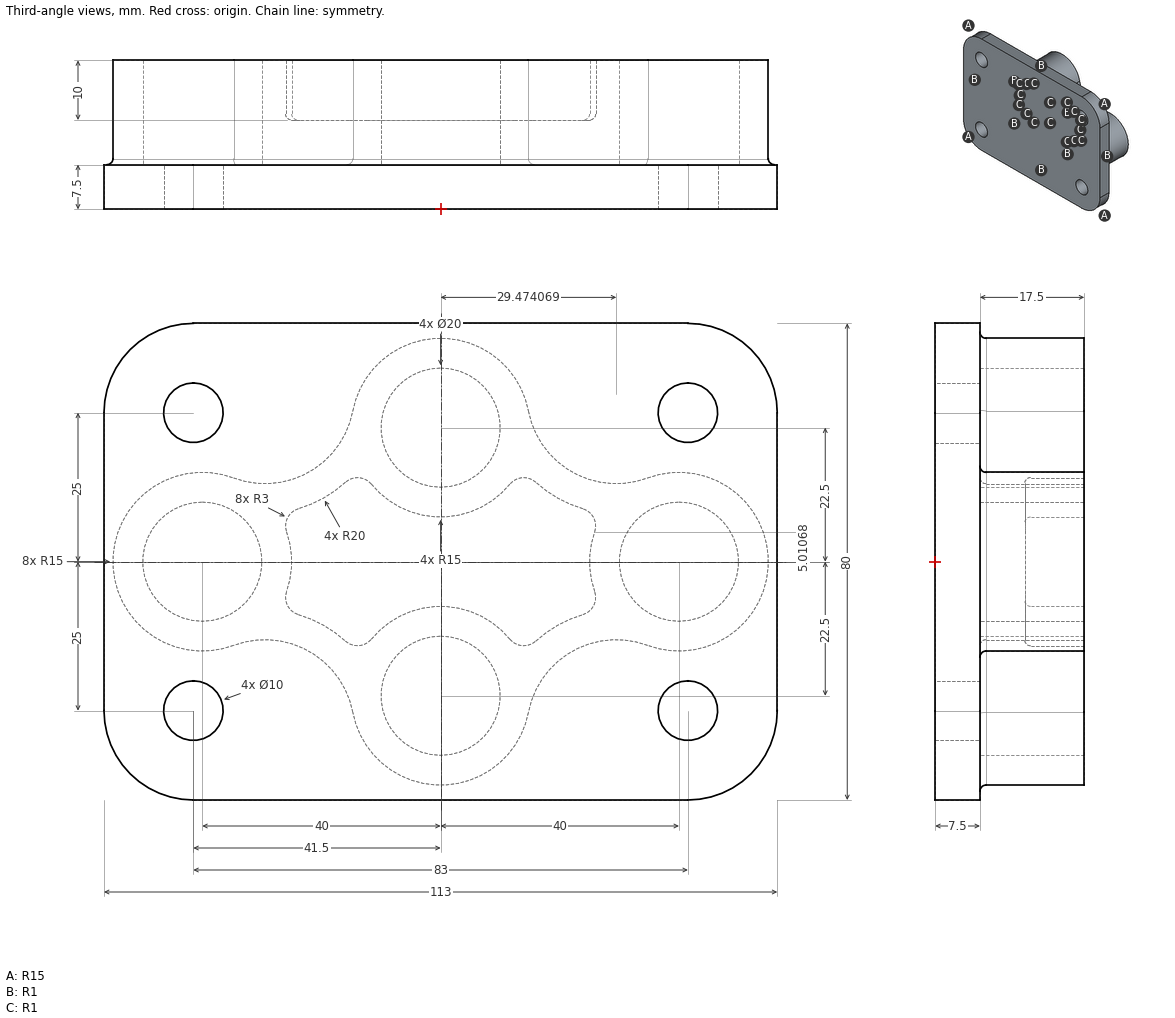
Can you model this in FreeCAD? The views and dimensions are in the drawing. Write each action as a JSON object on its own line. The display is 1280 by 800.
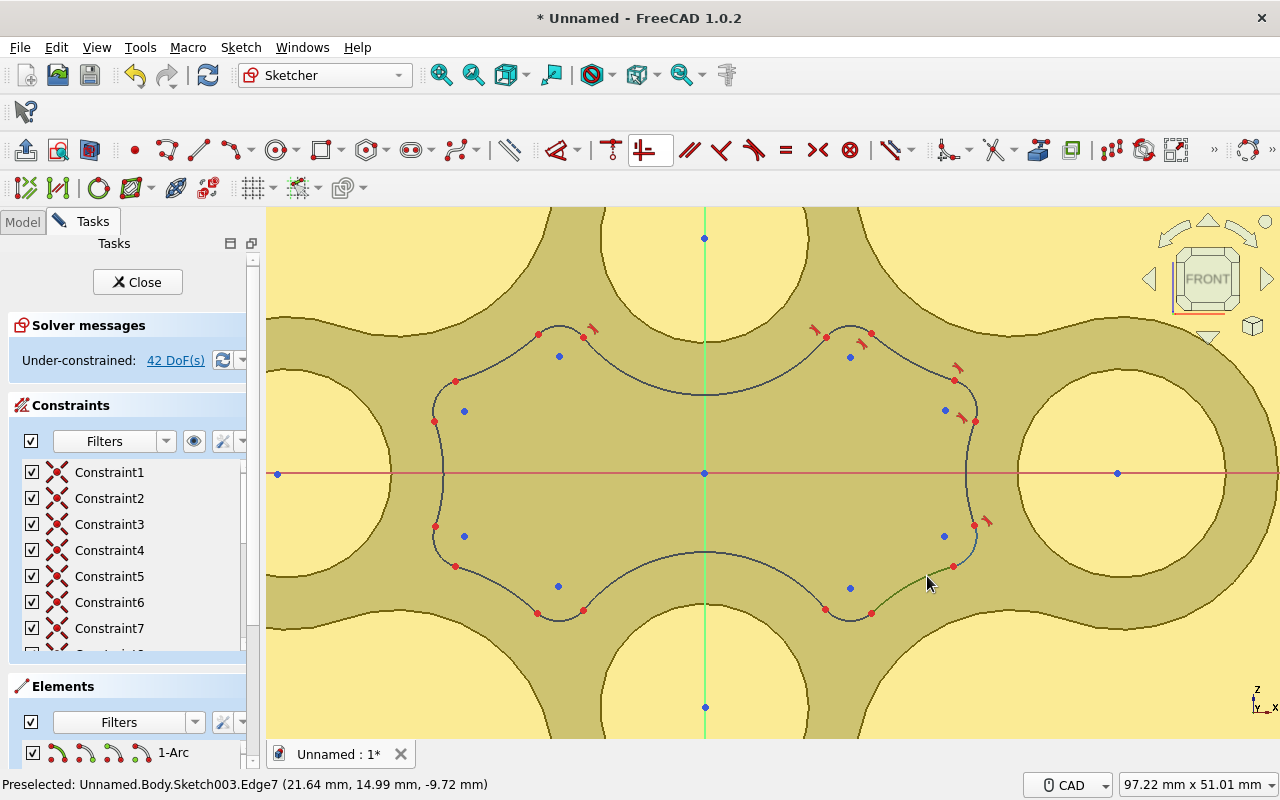
{"action": "key", "text": "t"}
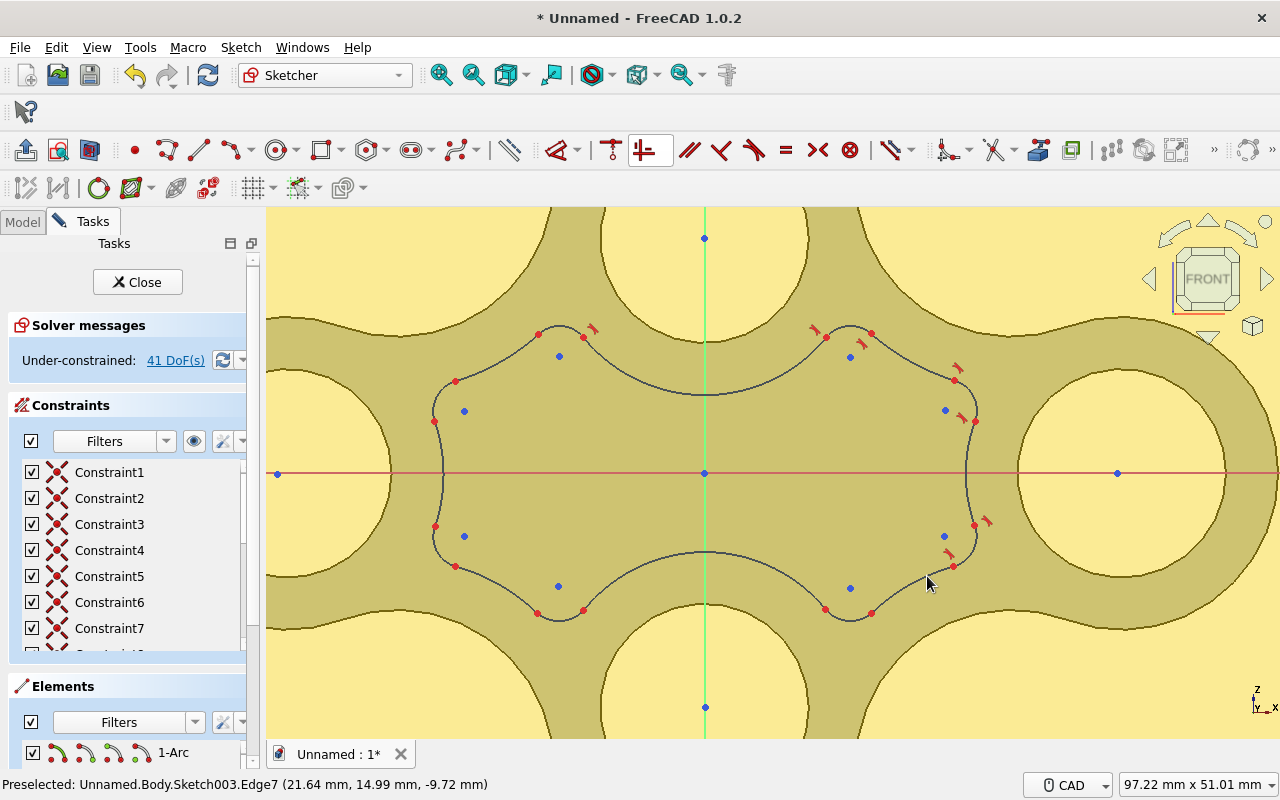
{"action": "left_click", "coordinate": [927, 576]}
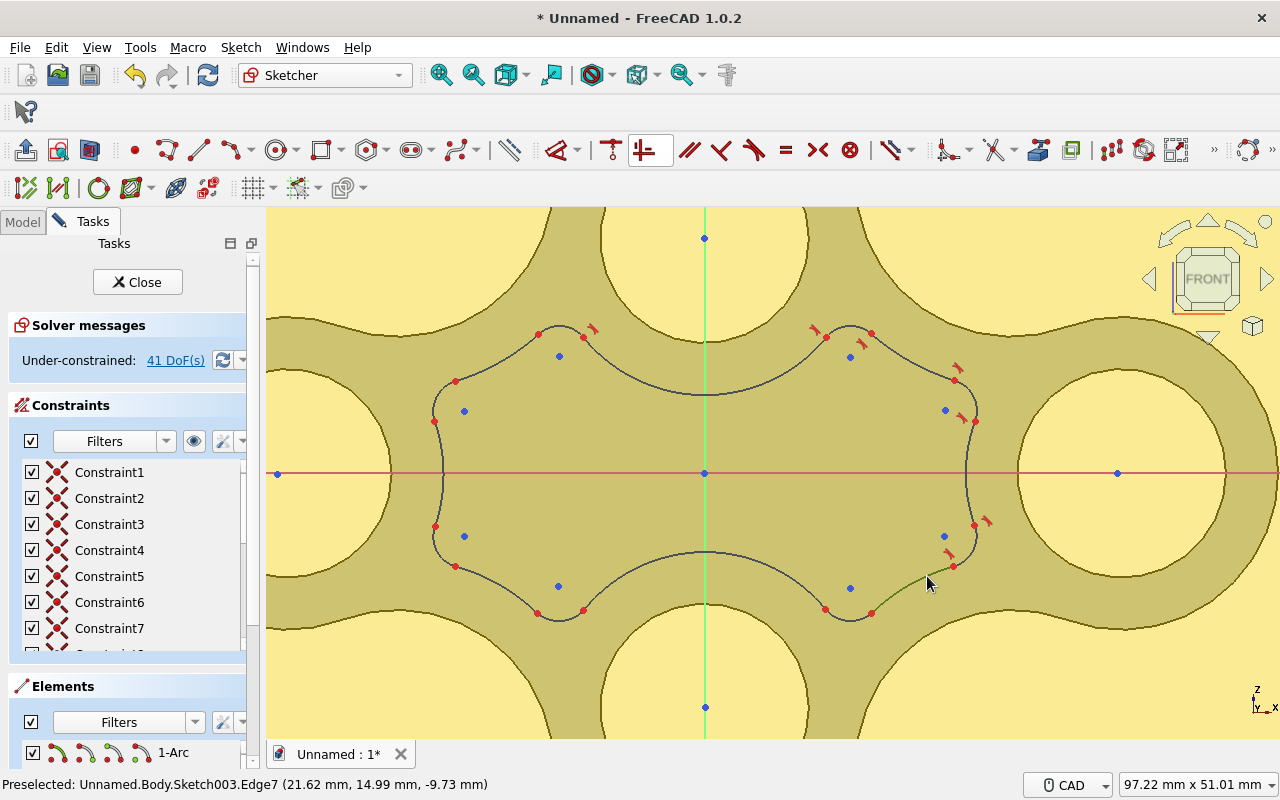
{"action": "left_click", "coordinate": [838, 618]}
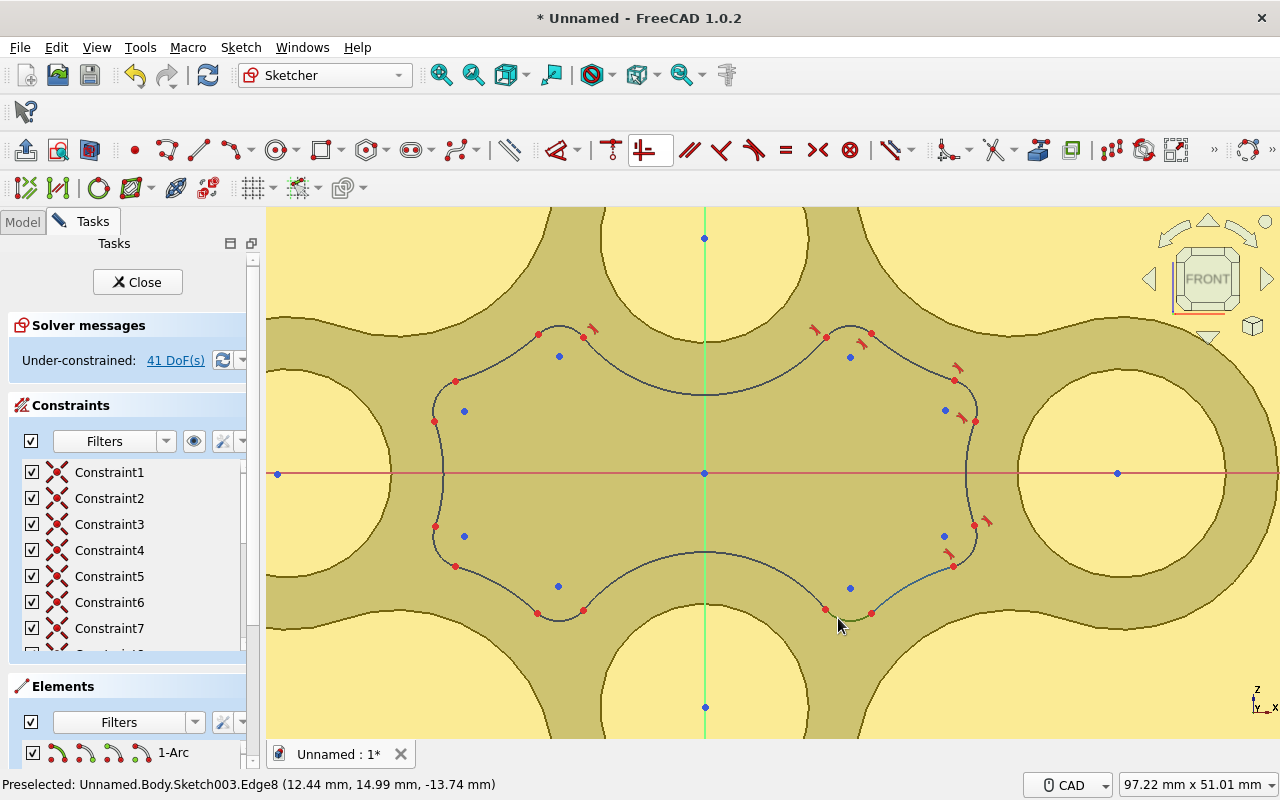
{"action": "key", "text": "t"}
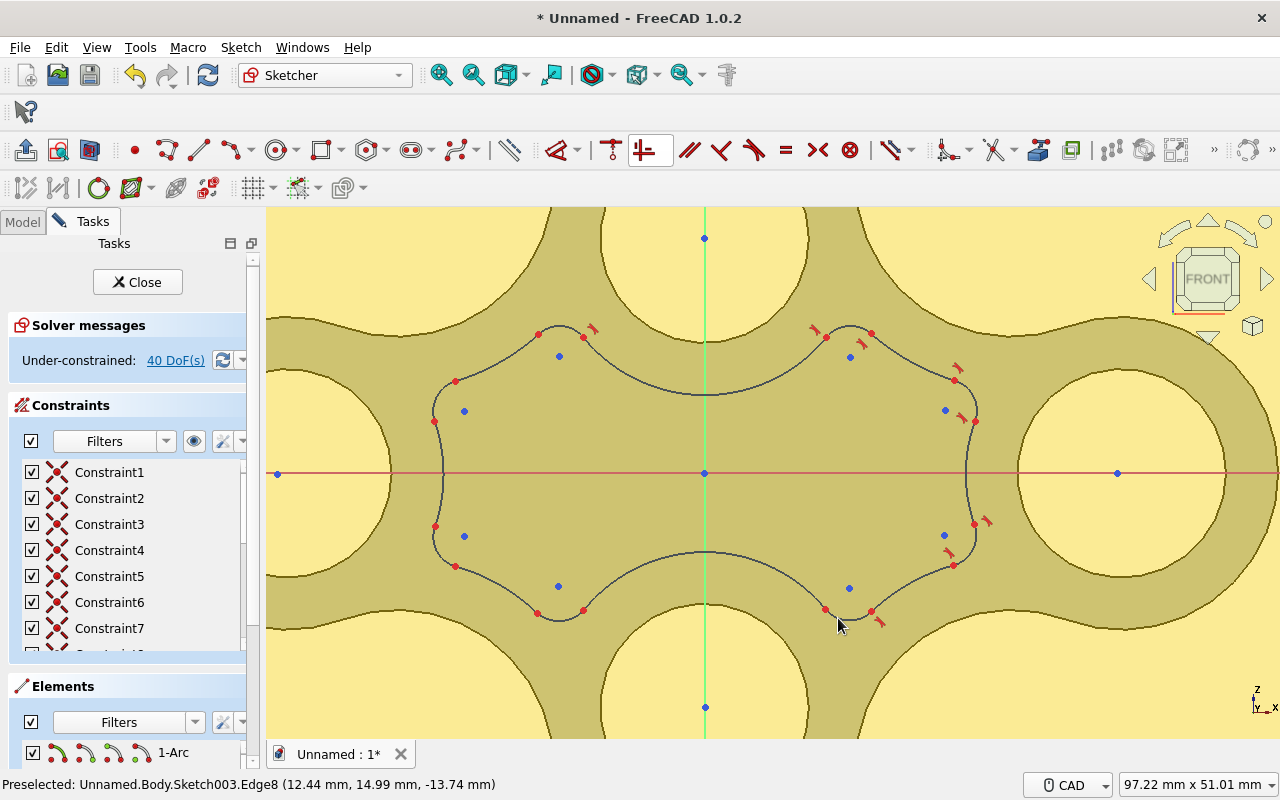
{"action": "left_click", "coordinate": [838, 618]}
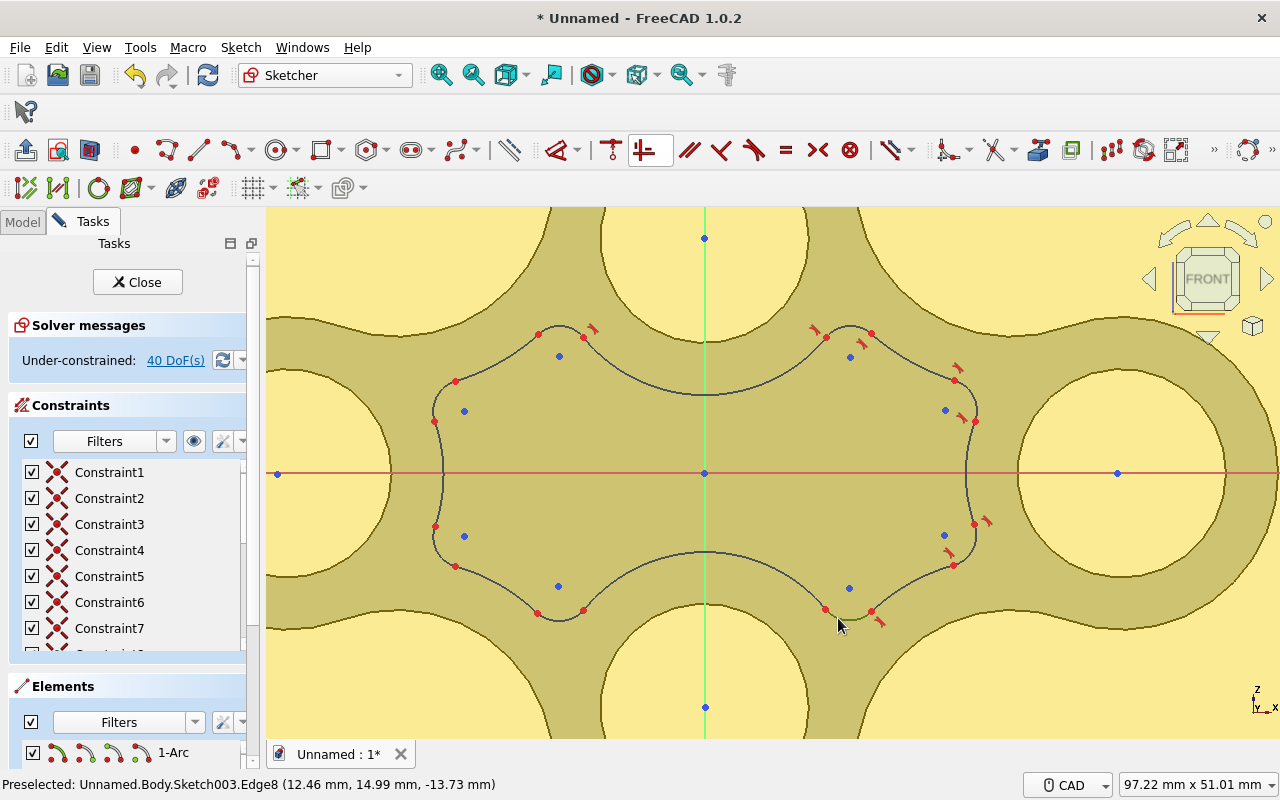
{"action": "left_click", "coordinate": [759, 562]}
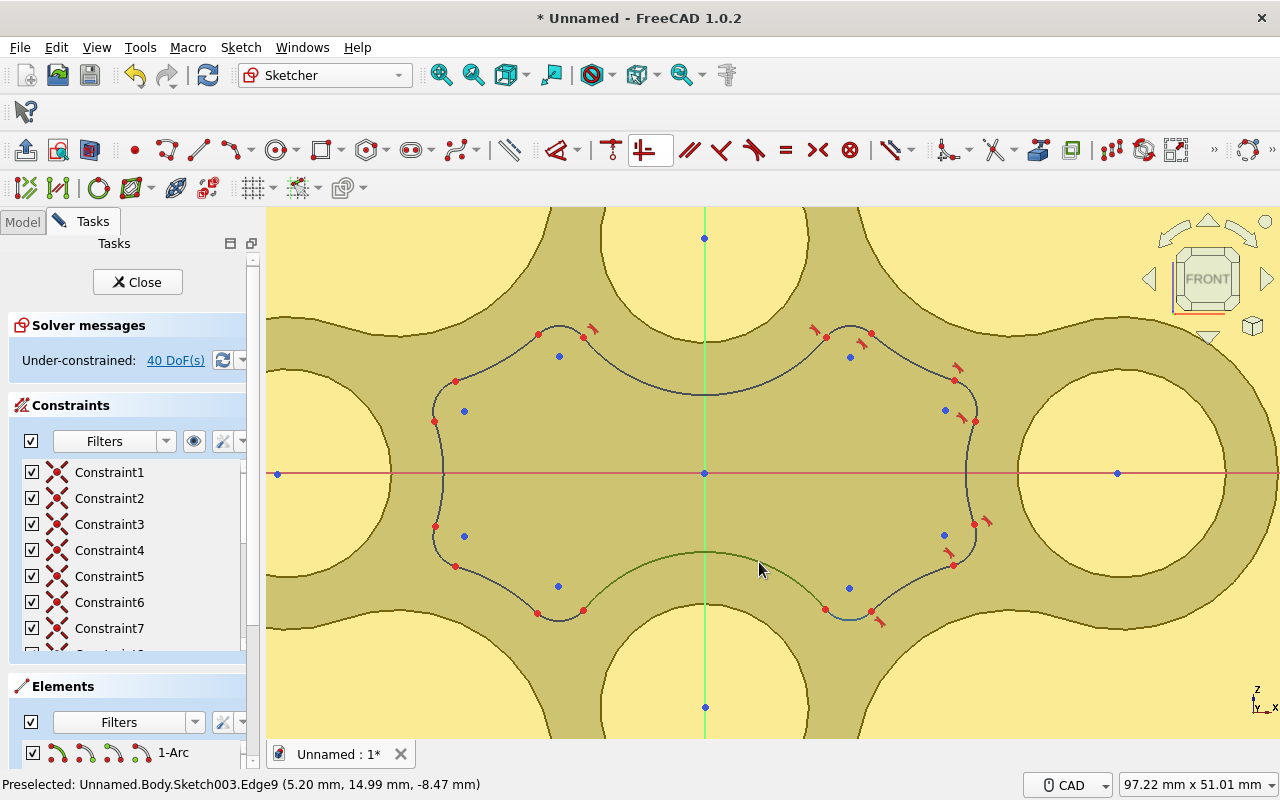
{"action": "key", "text": "t"}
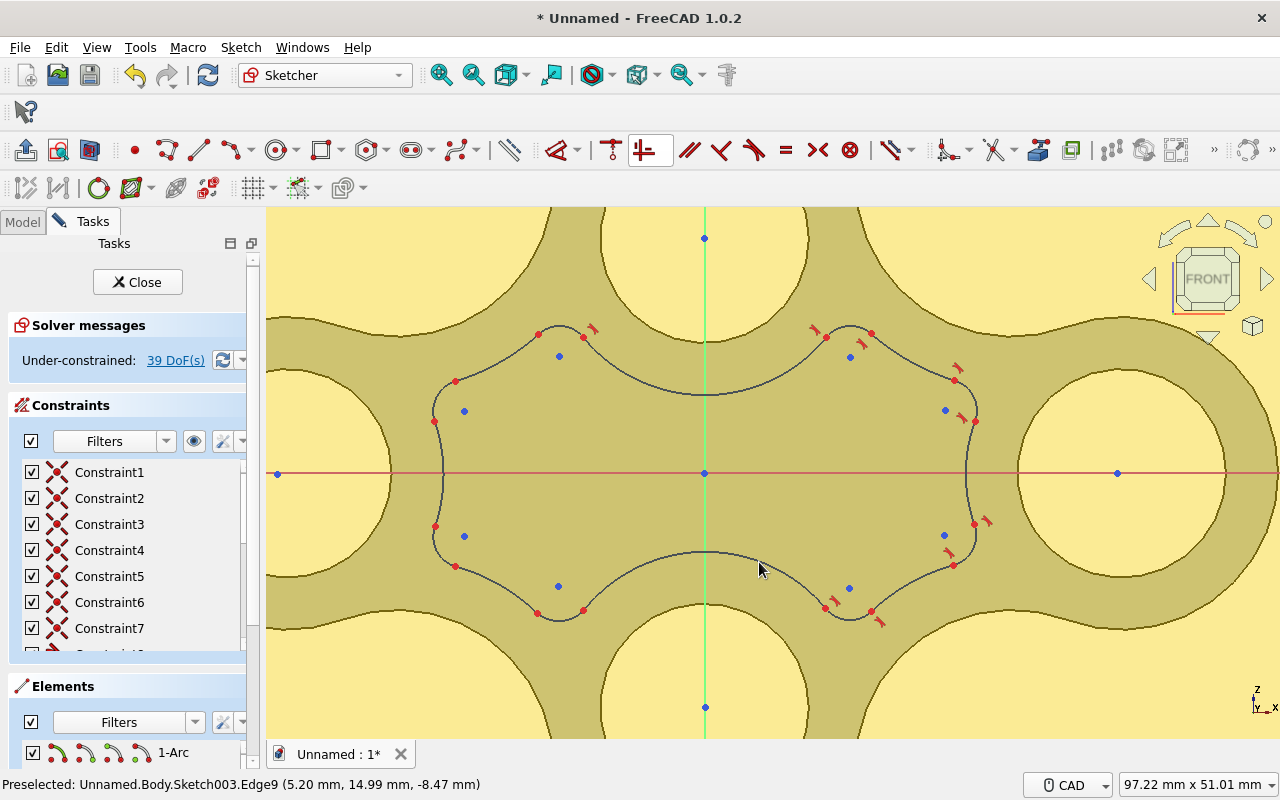
{"action": "left_click", "coordinate": [759, 561]}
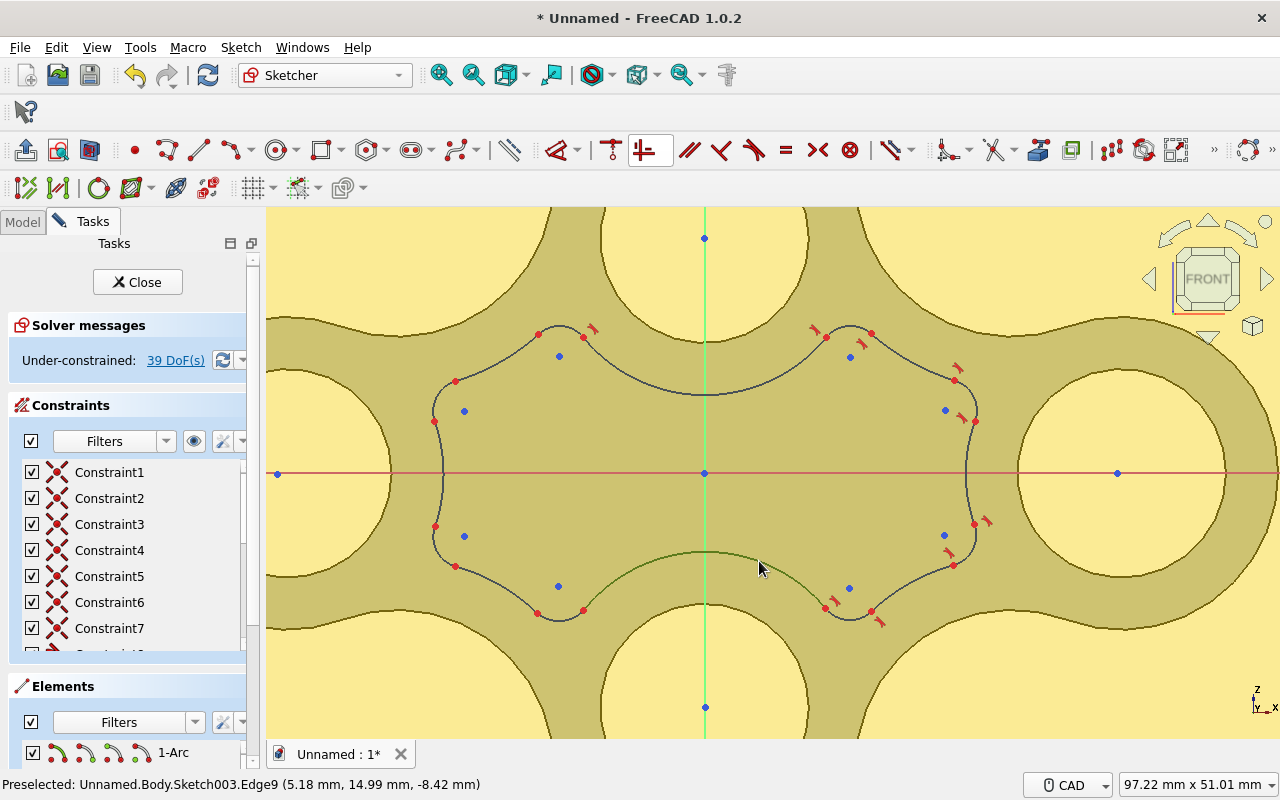
{"action": "left_click", "coordinate": [551, 620]}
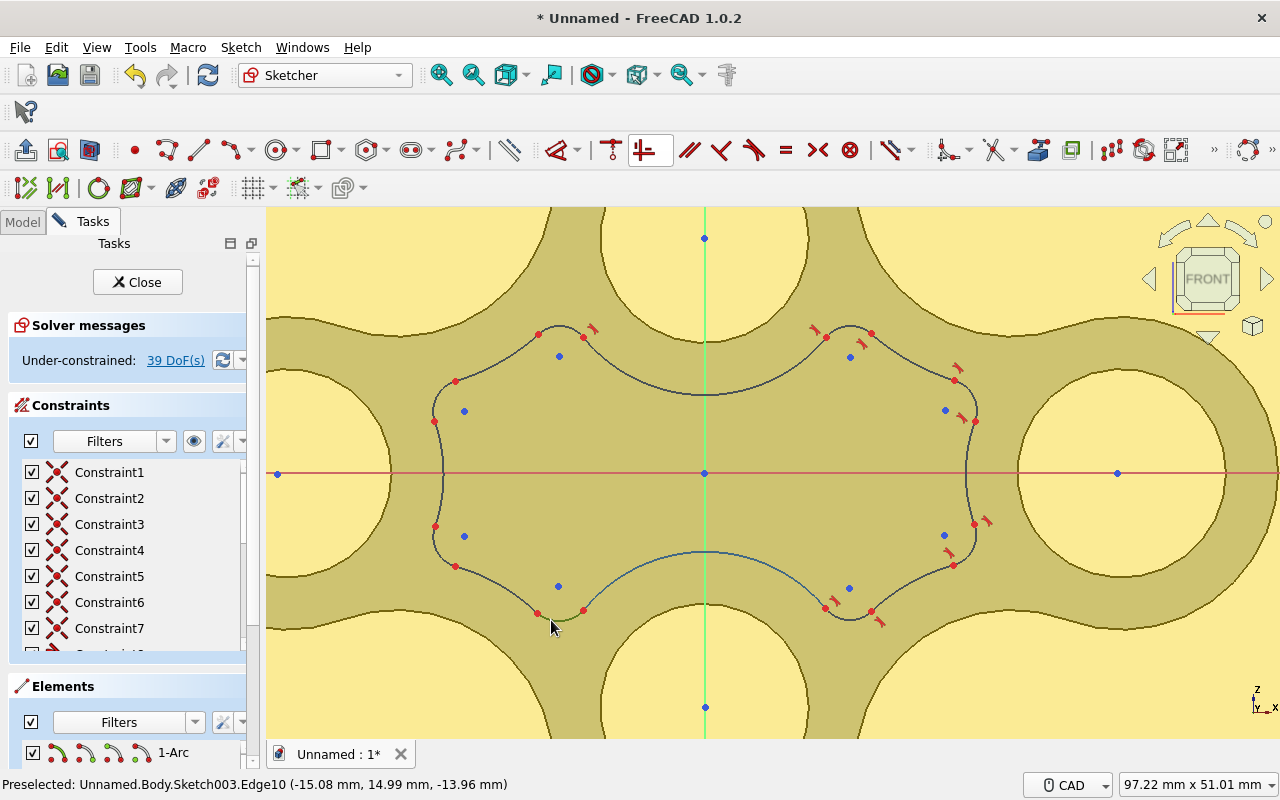
{"action": "left_click", "coordinate": [754, 150]}